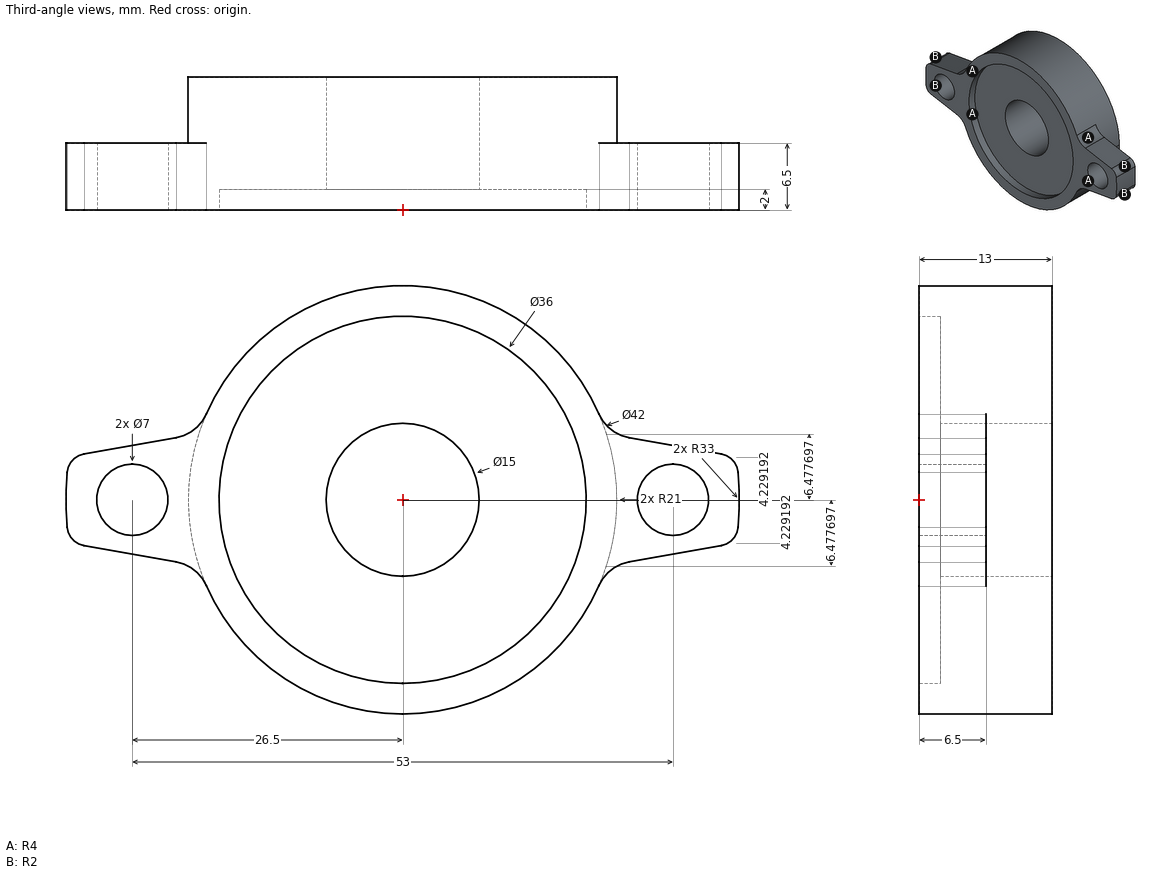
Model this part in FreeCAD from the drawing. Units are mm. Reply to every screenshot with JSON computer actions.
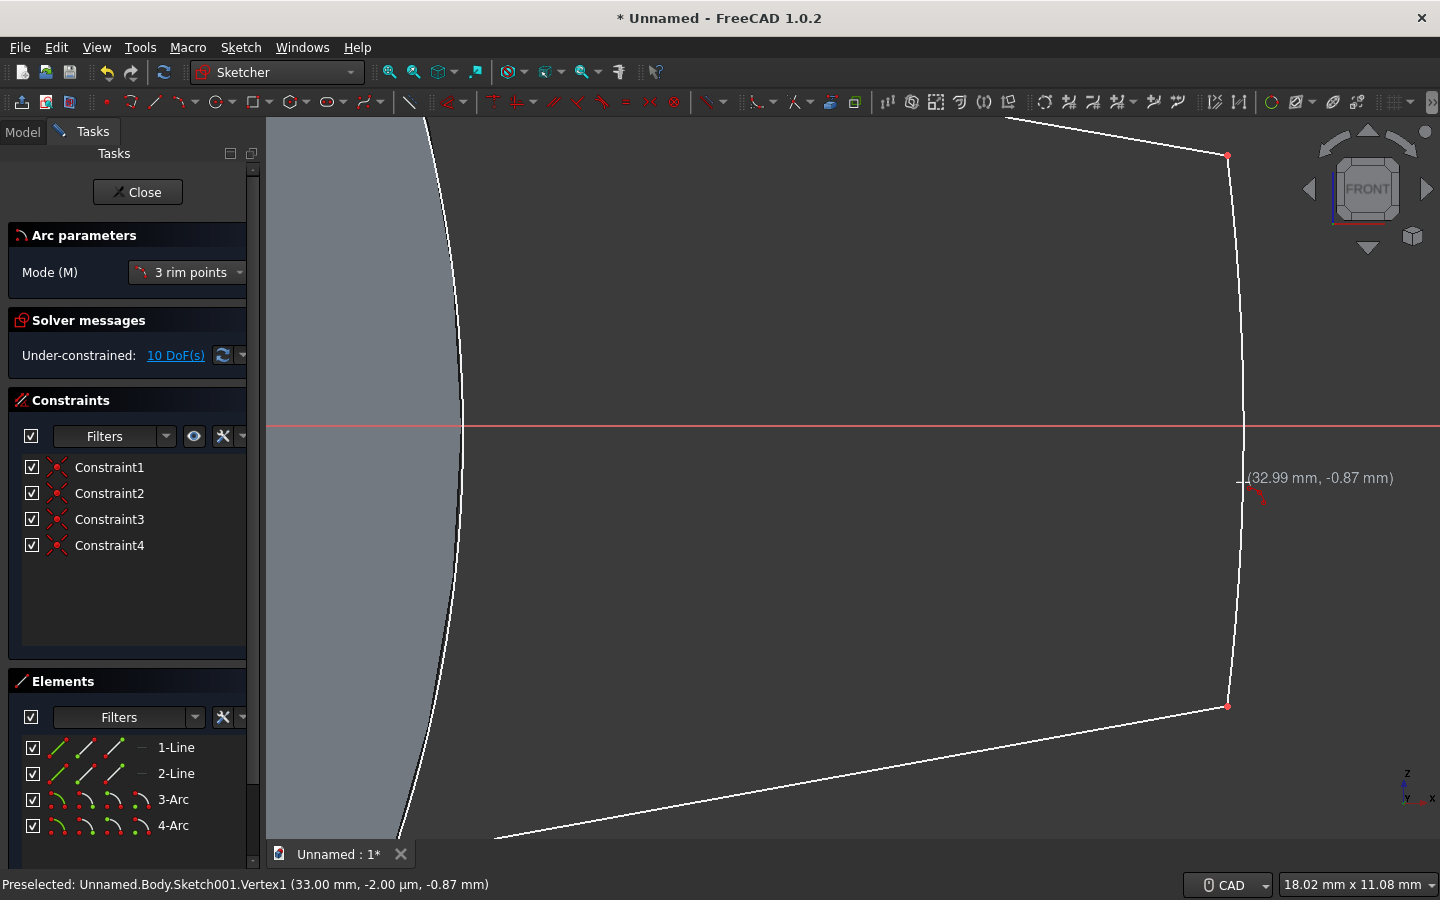
{"action": "left_click", "coordinate": [156, 102]}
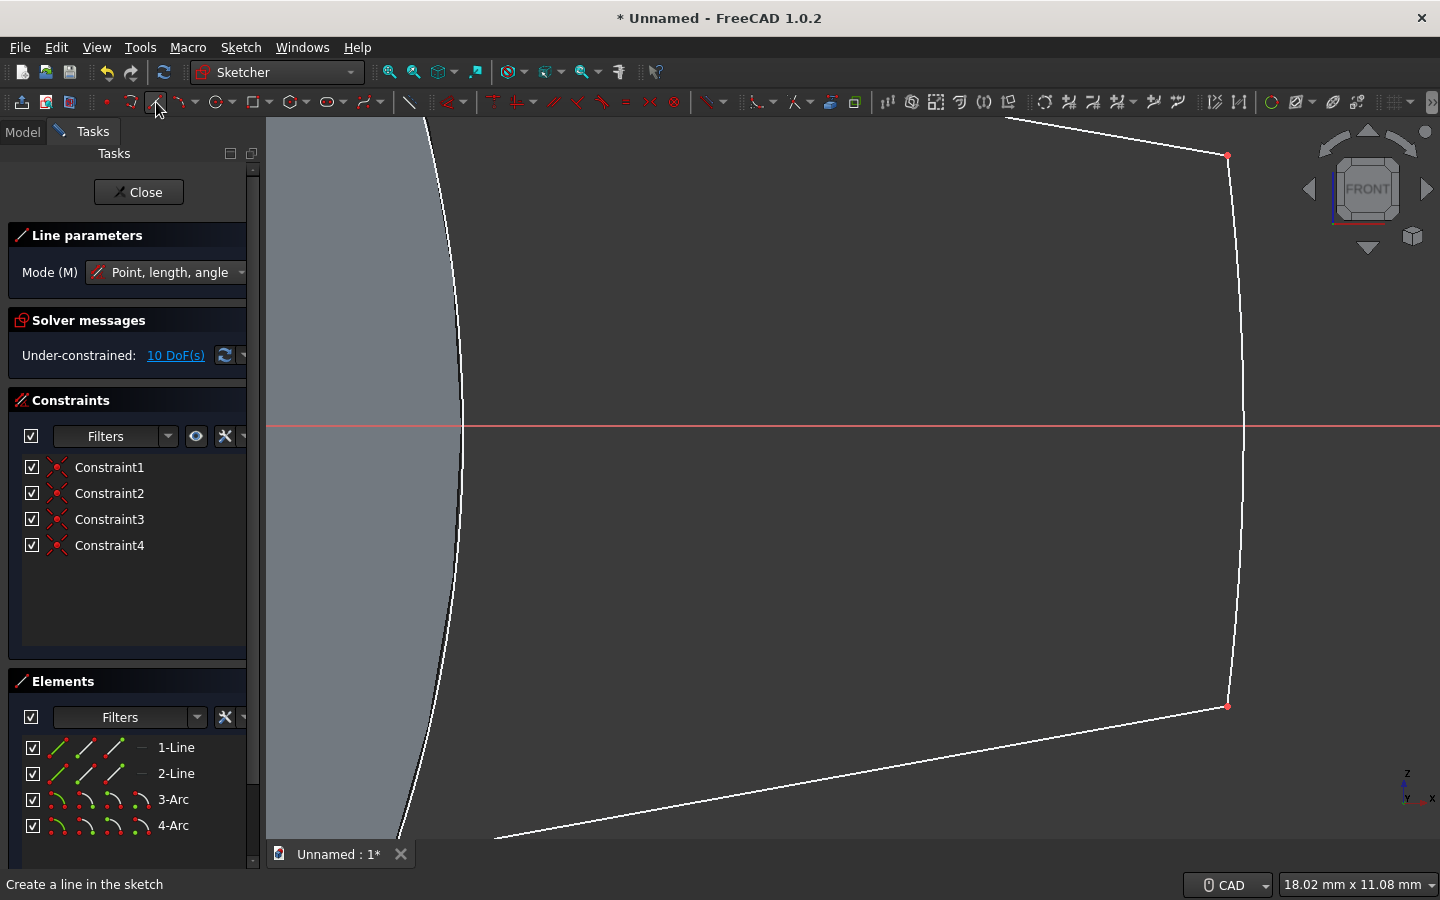
{"action": "scroll", "coordinate": [1119, 488], "scroll_direction": "down", "scroll_amount": 9}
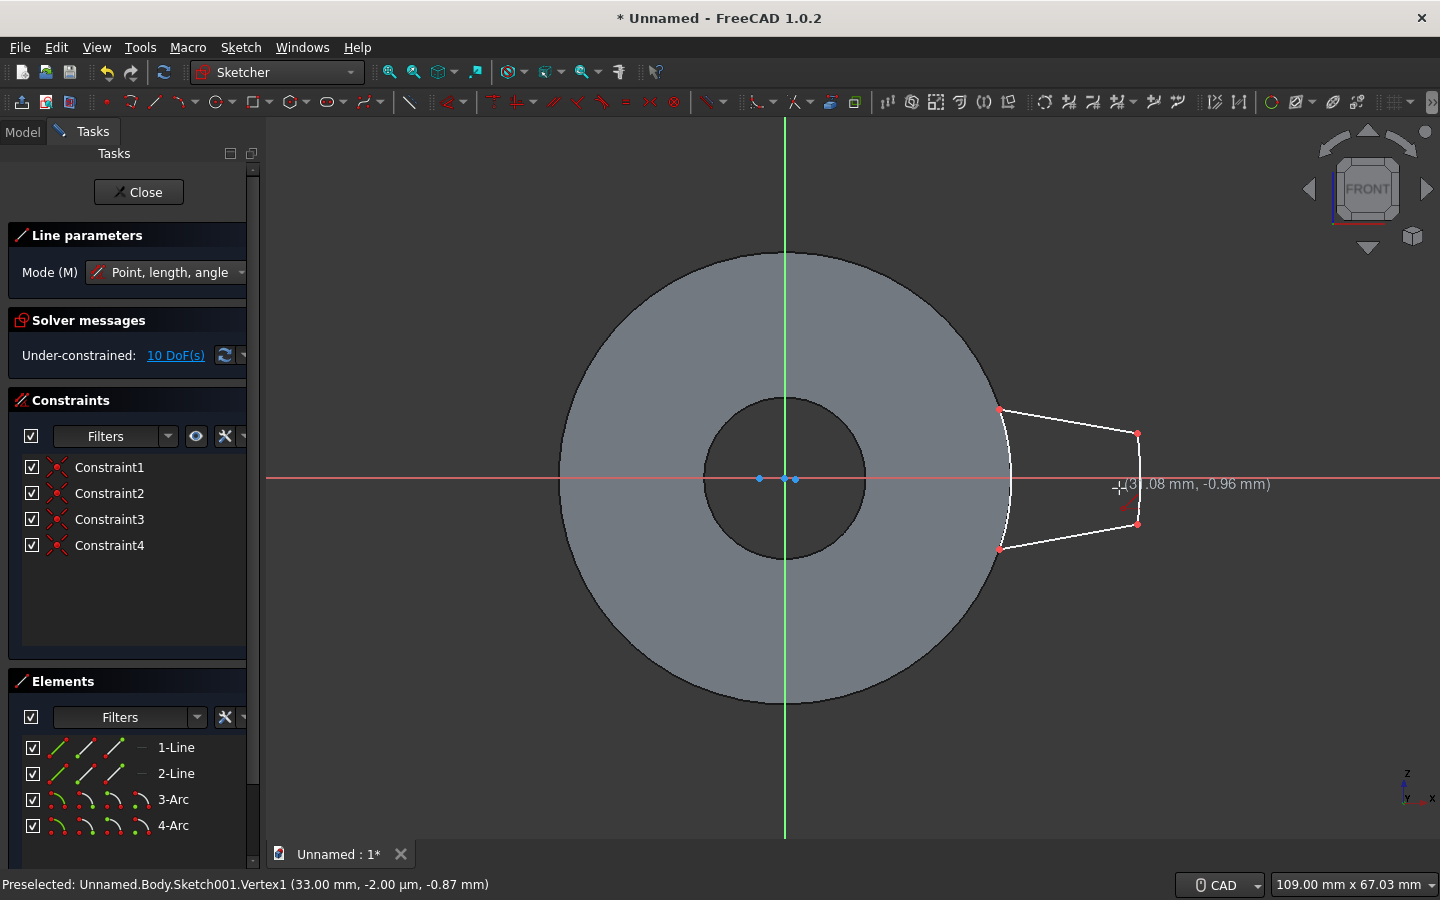
{"action": "left_click", "coordinate": [432, 524]}
{"action": "left_click", "coordinate": [570, 548]}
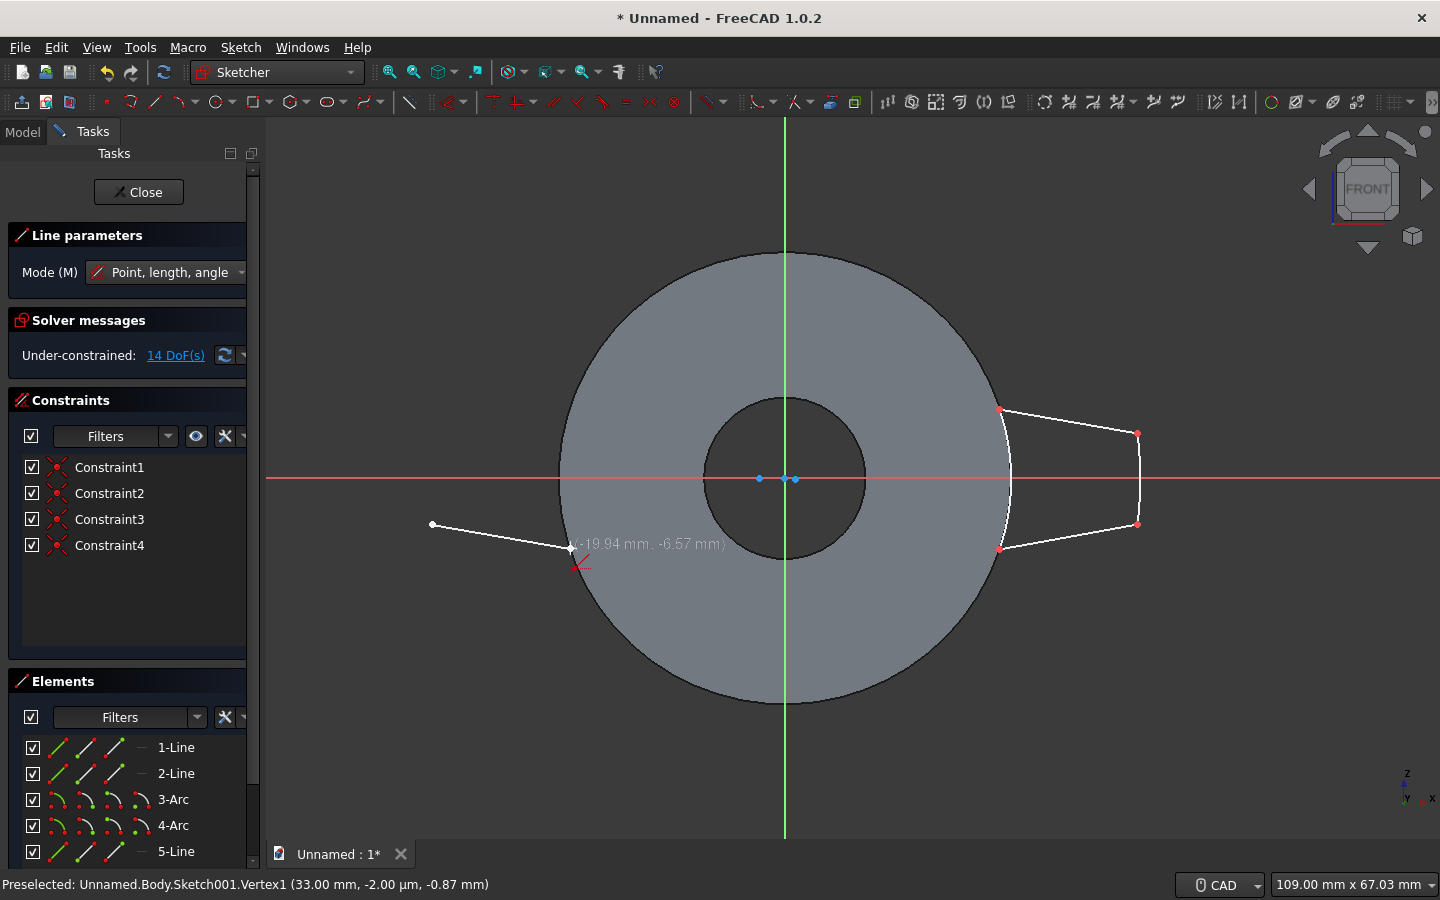
{"action": "left_click", "coordinate": [570, 408]}
{"action": "left_click", "coordinate": [432, 433]}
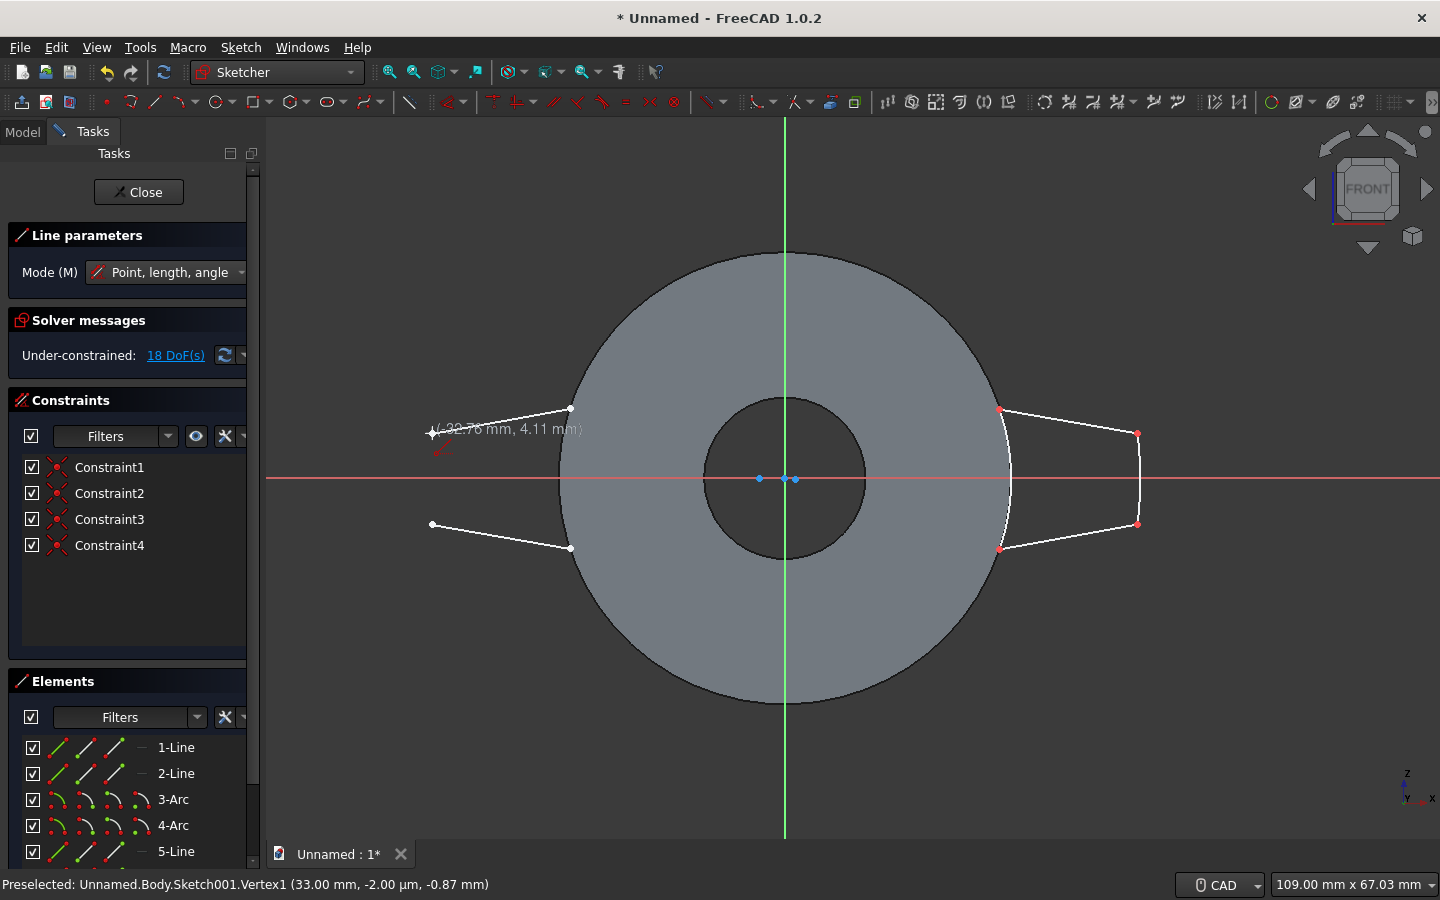
{"action": "left_click", "coordinate": [180, 102]}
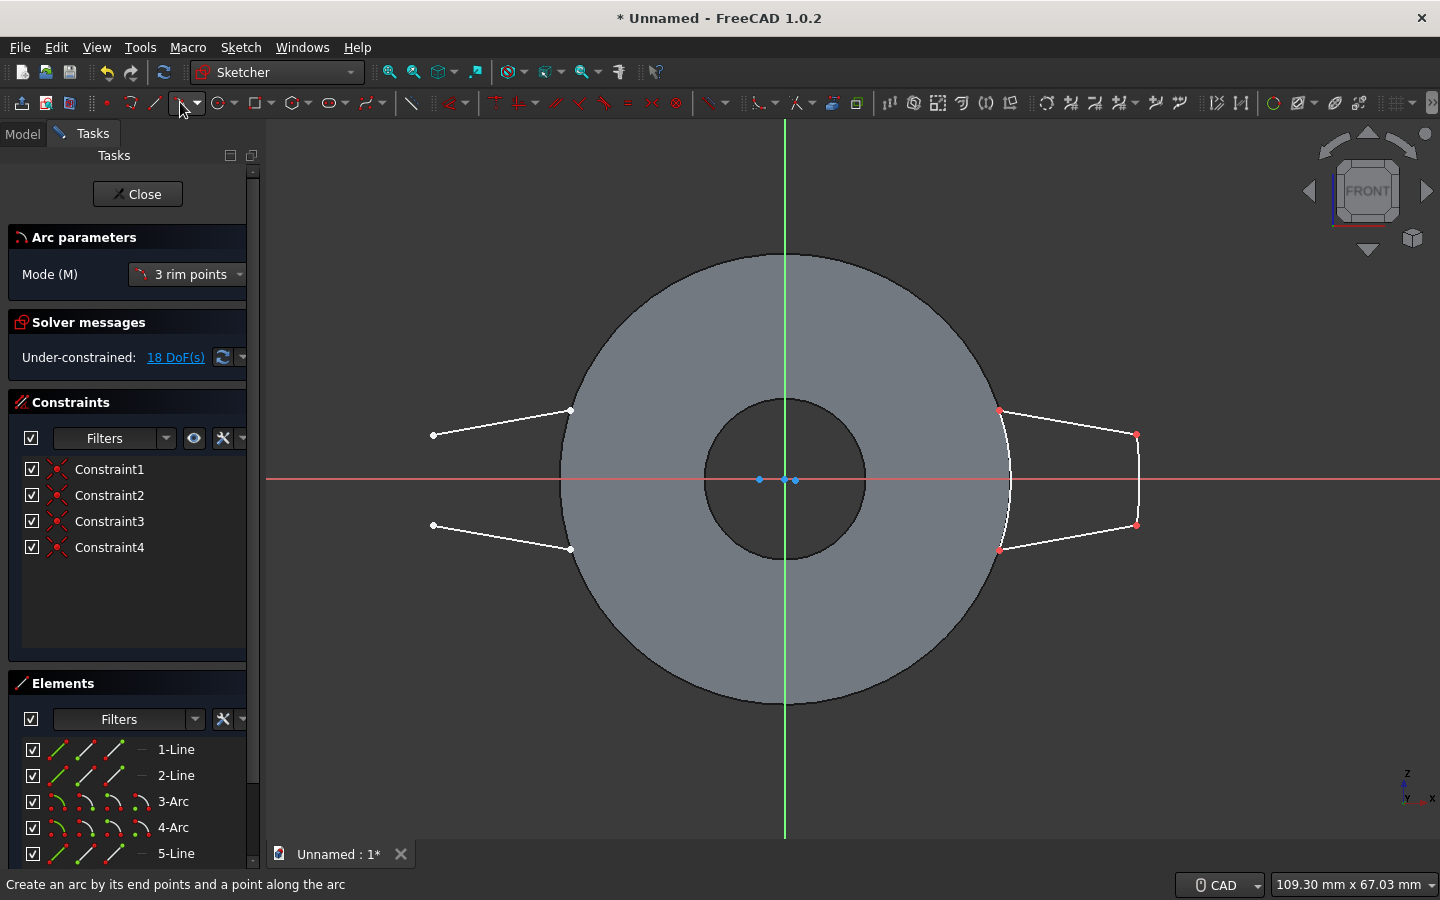
{"action": "left_click", "coordinate": [571, 550]}
{"action": "left_click", "coordinate": [571, 410]}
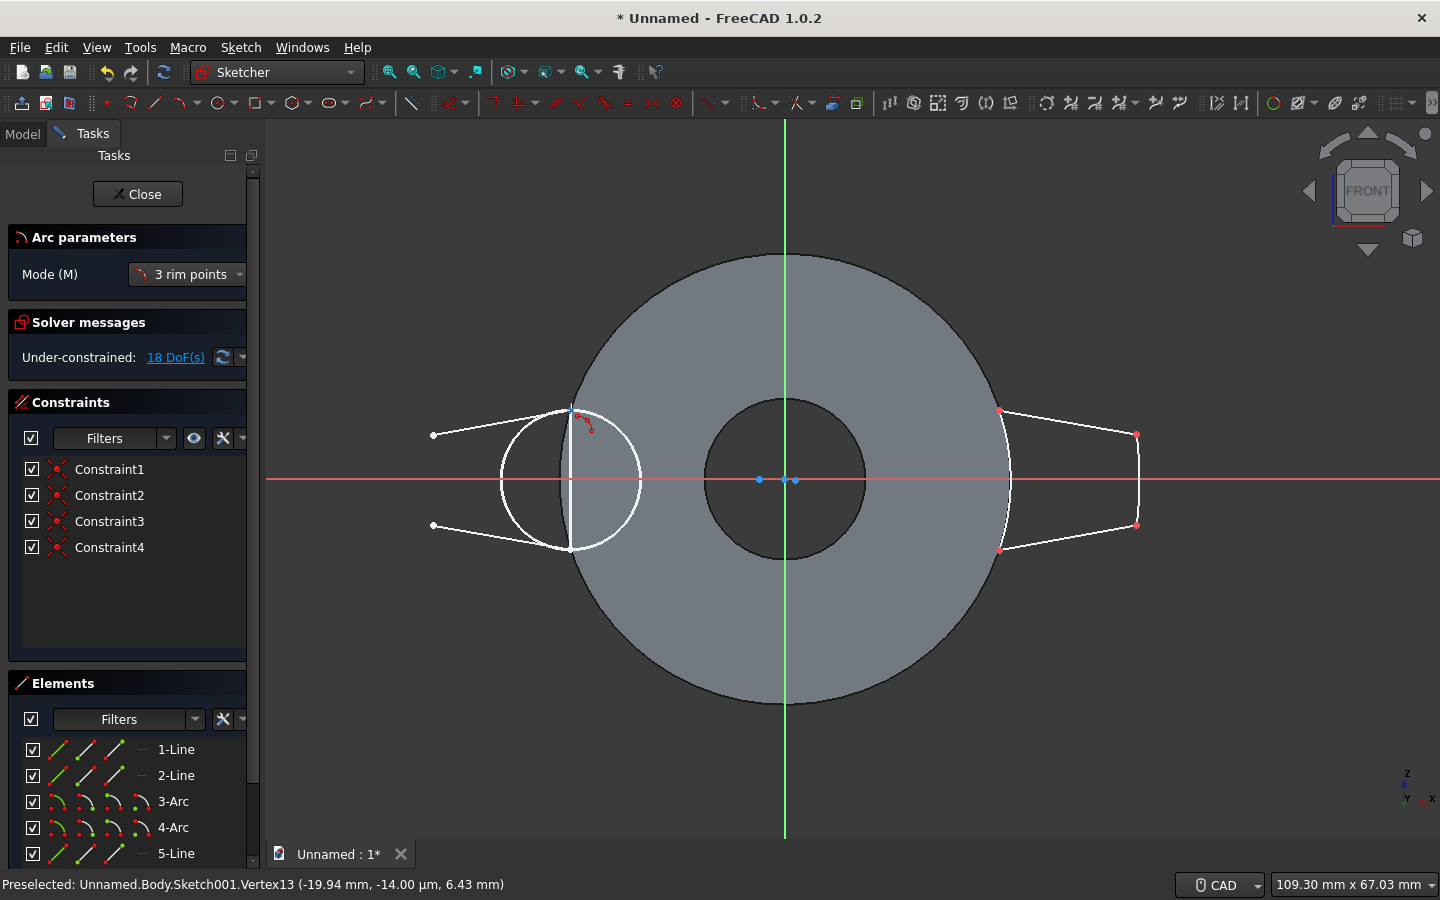
{"action": "scroll", "coordinate": [560, 465], "scroll_direction": "up", "scroll_amount": 3}